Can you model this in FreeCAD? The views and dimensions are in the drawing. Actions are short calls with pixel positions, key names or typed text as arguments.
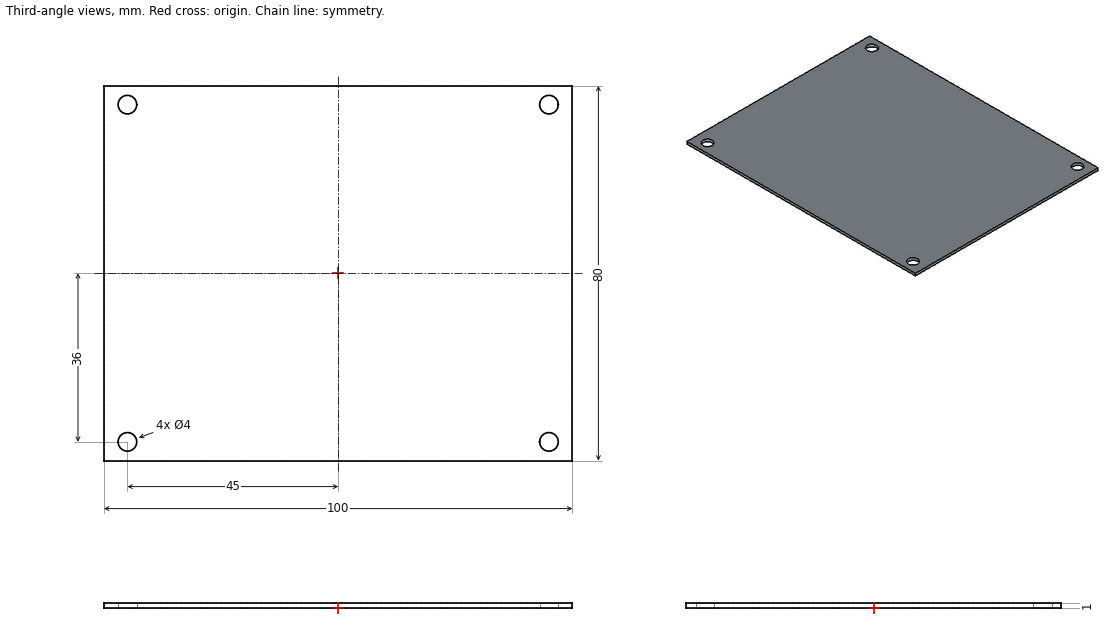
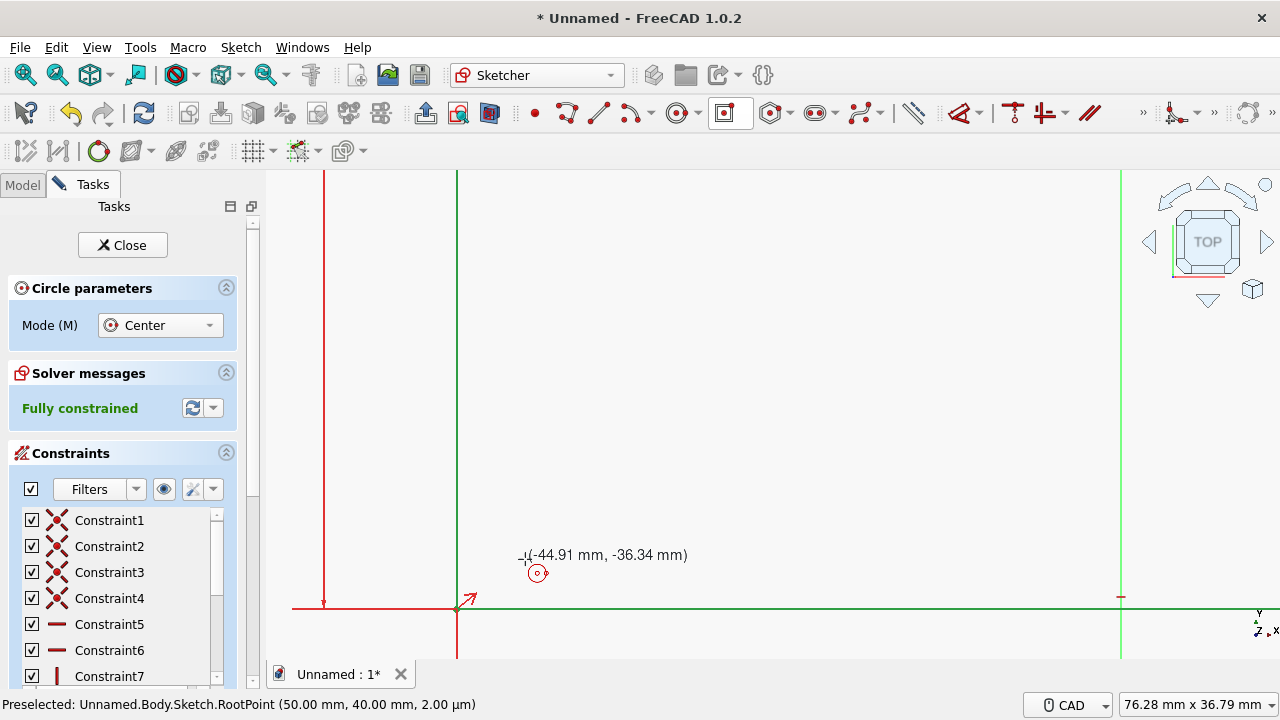
click(523, 556)
move(542, 537)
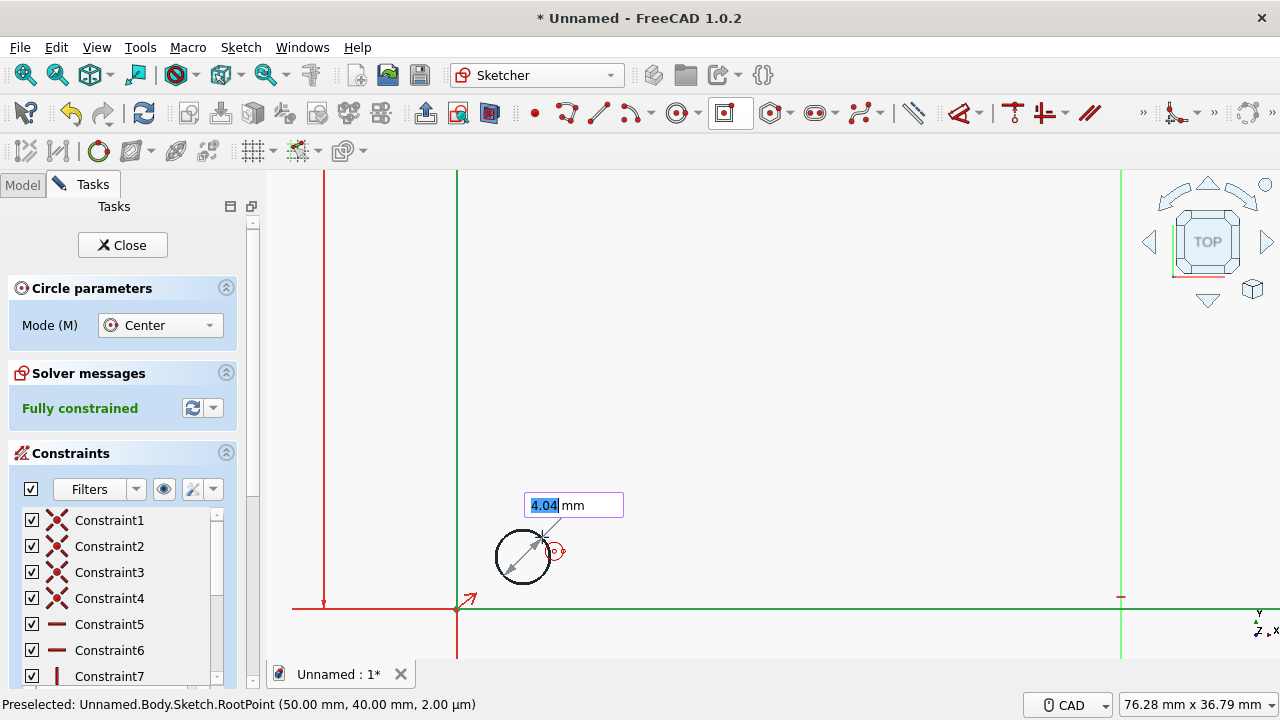
text(4)
key(Return)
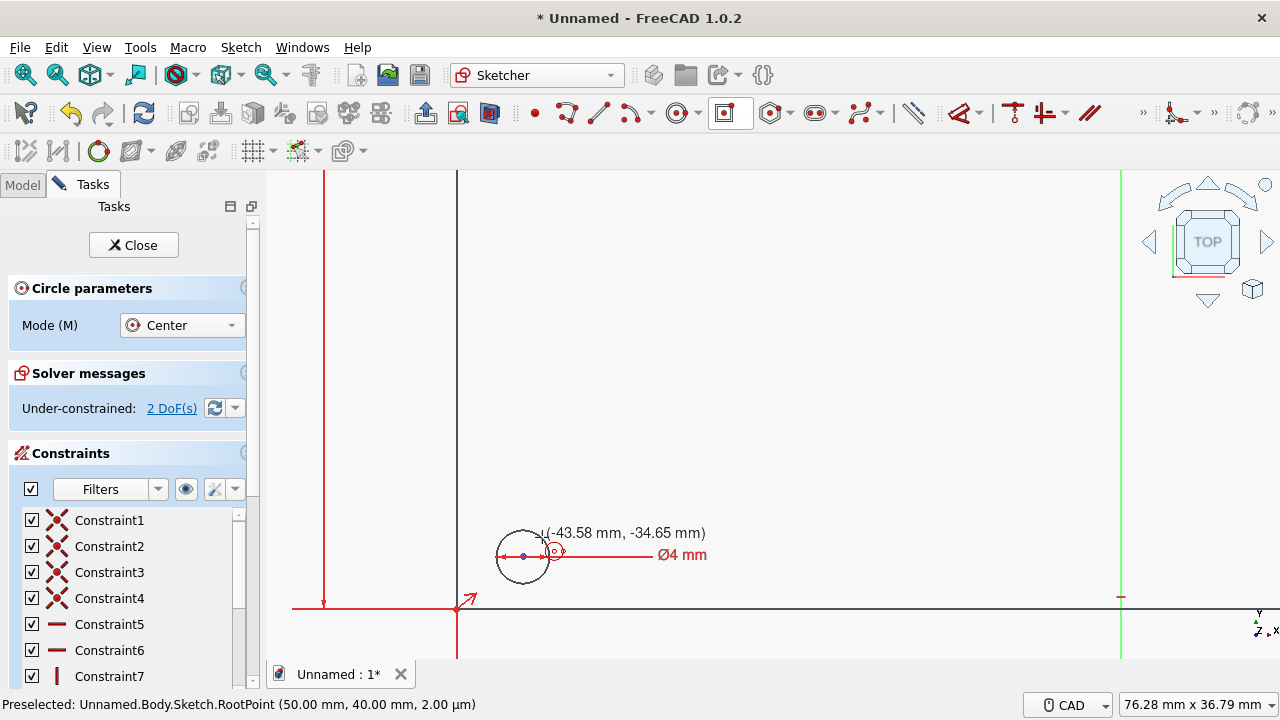
scroll(525, 560, down, 6)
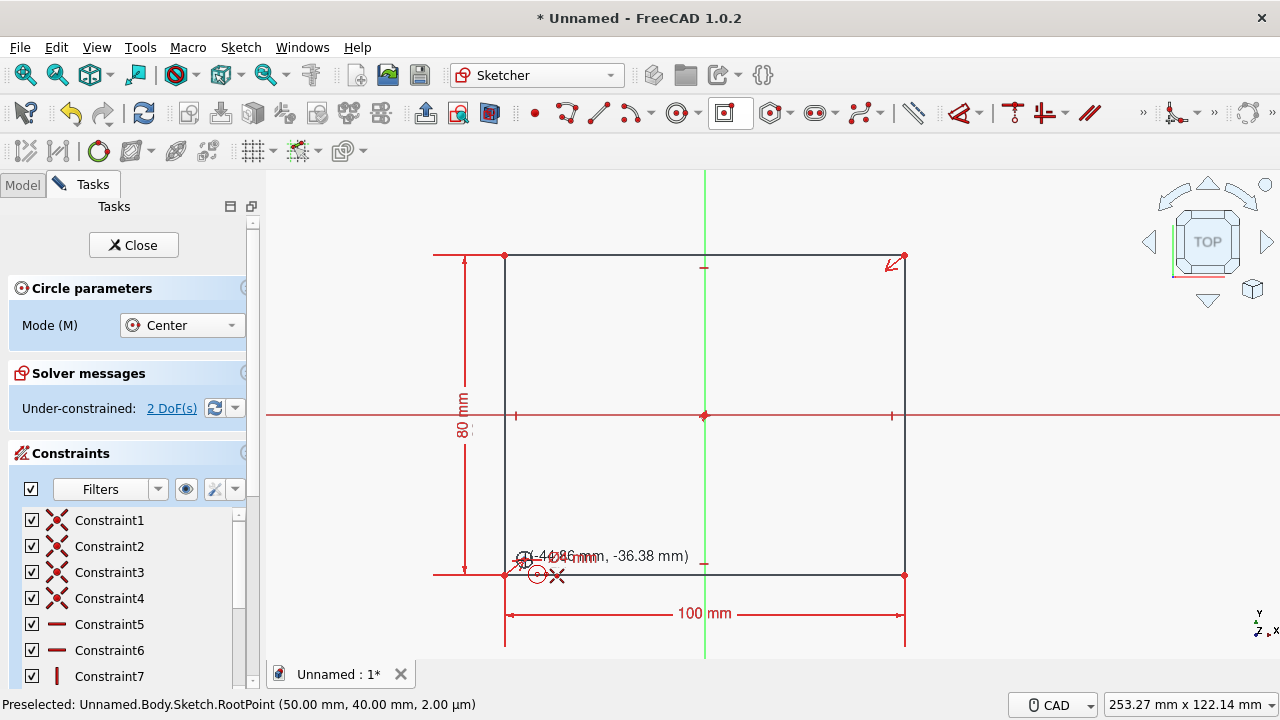
scroll(885, 559, up, 6)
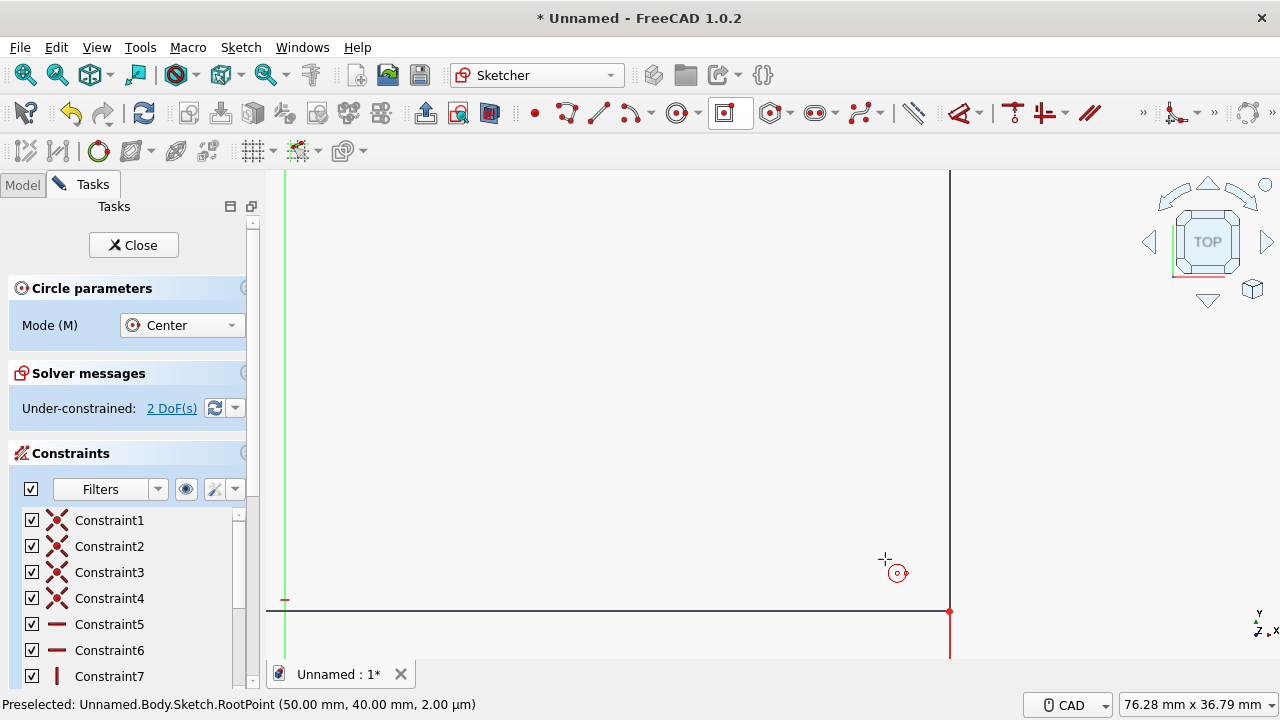
click(883, 558)
move(902, 539)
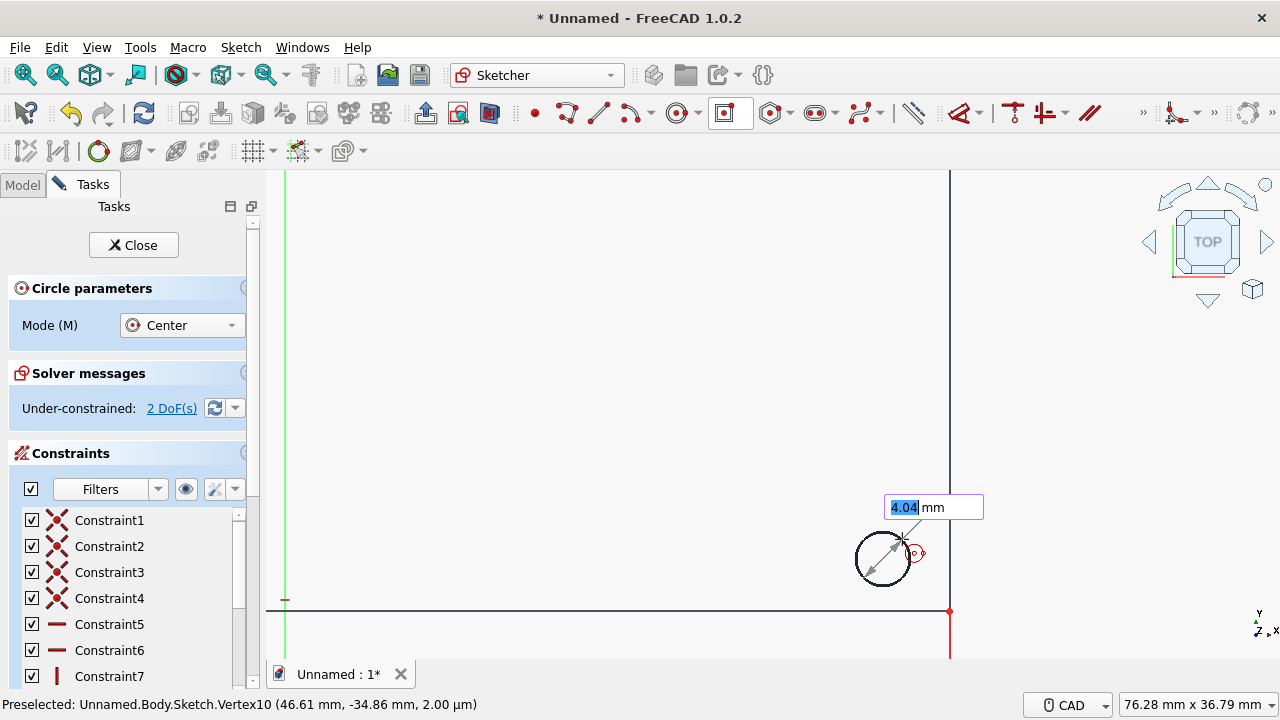
text(4)
key(Return)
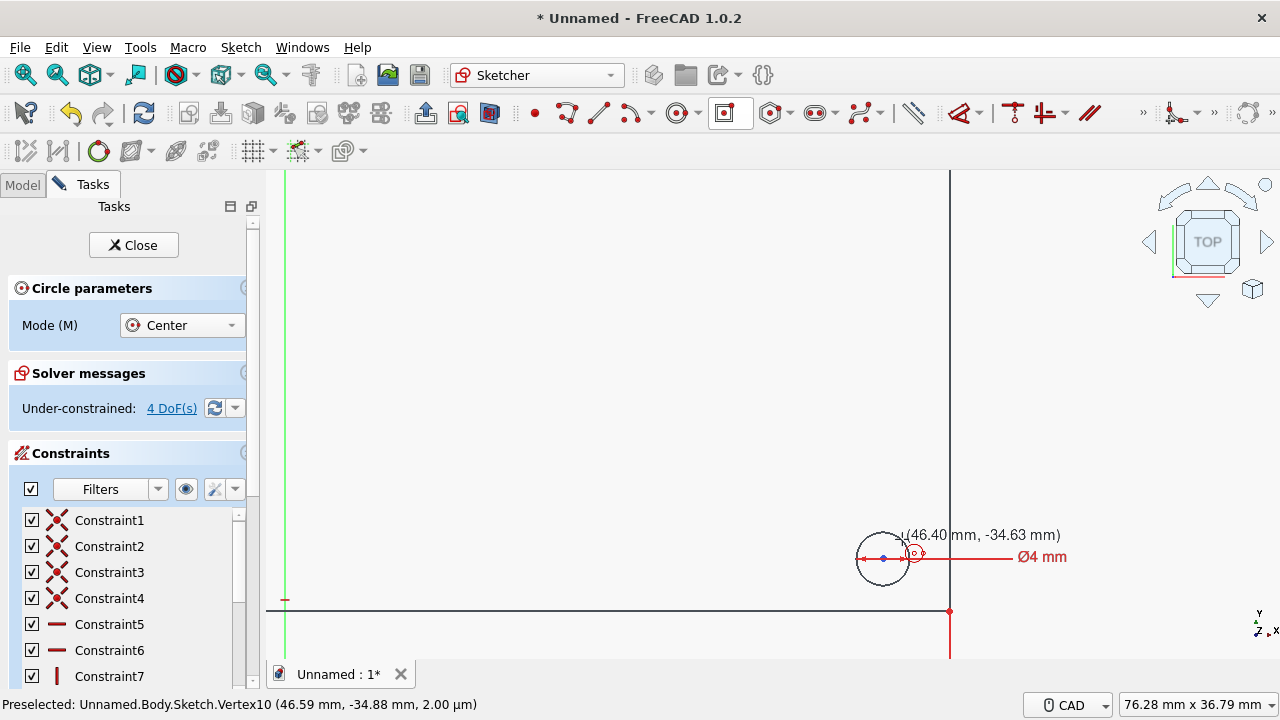
scroll(885, 559, down, 6)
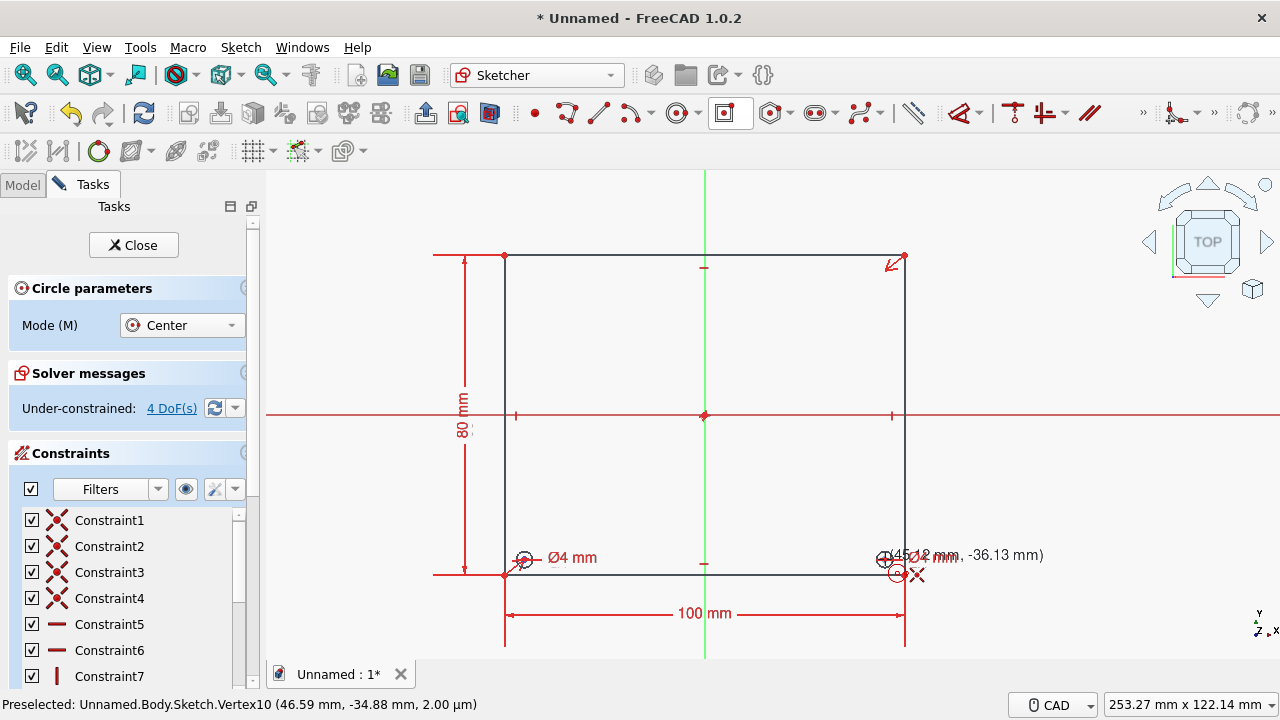
scroll(525, 271, up, 6)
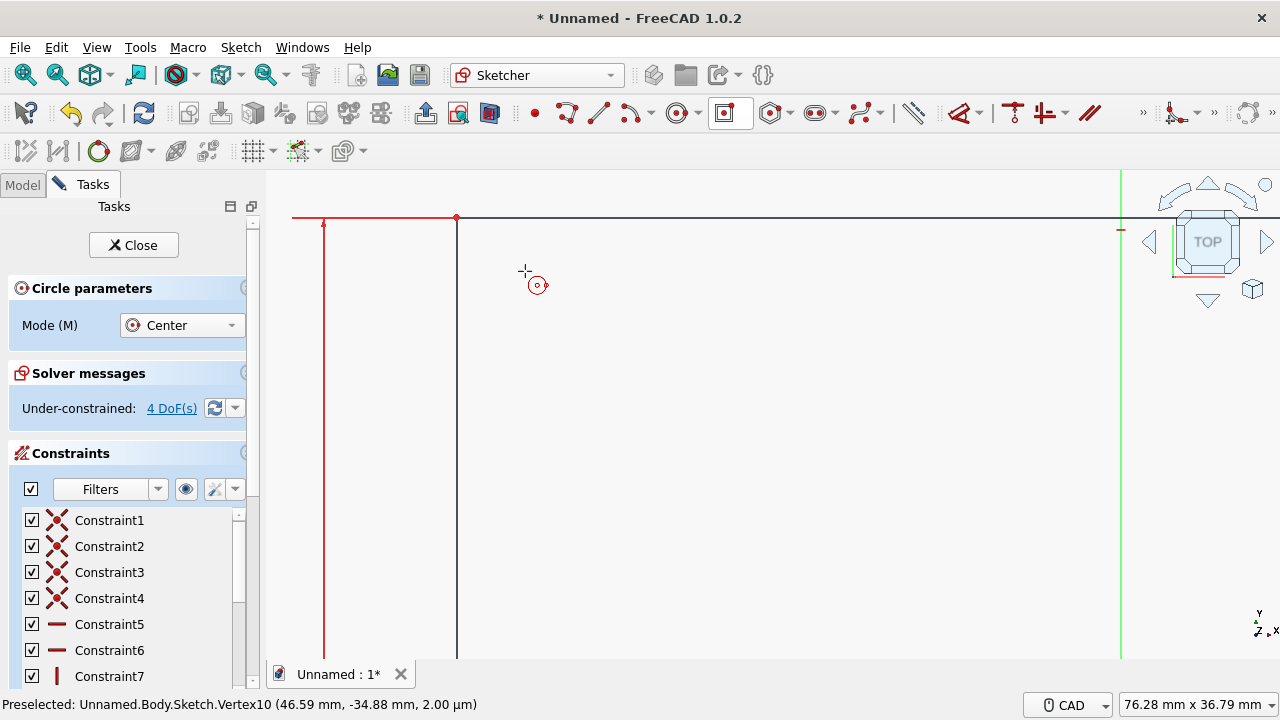
click(523, 271)
move(542, 252)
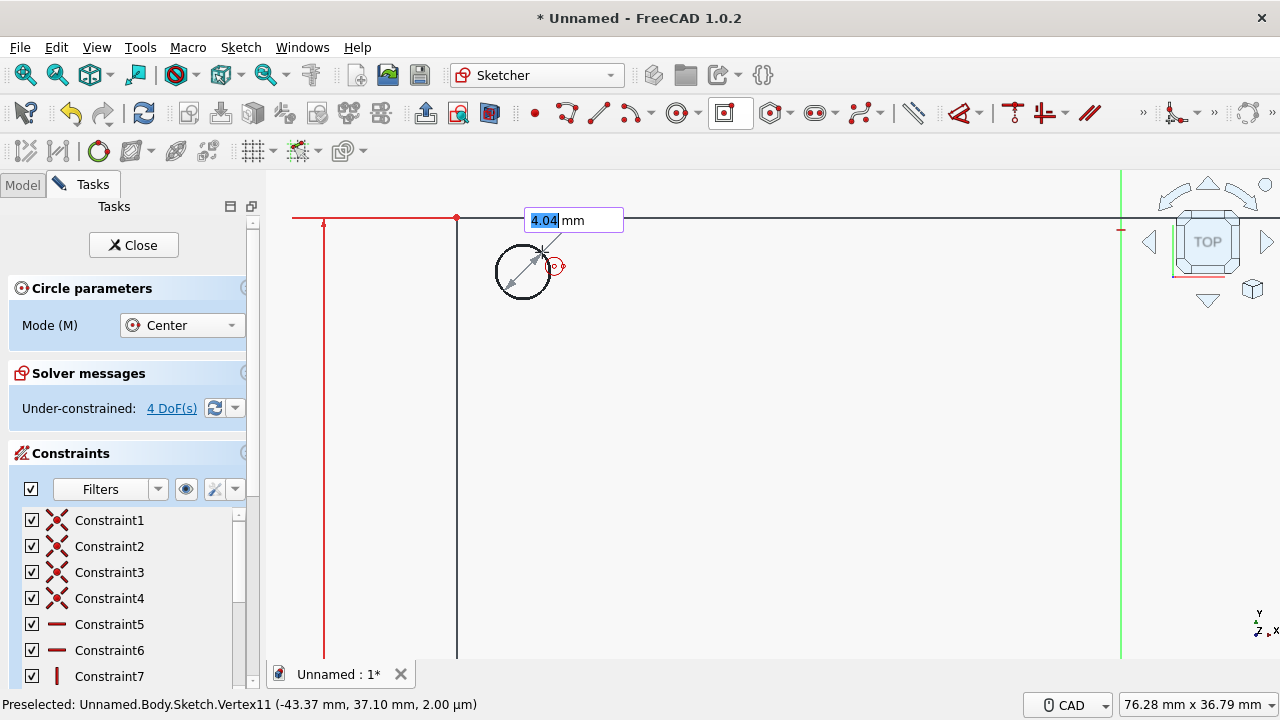
text(4)
key(Return)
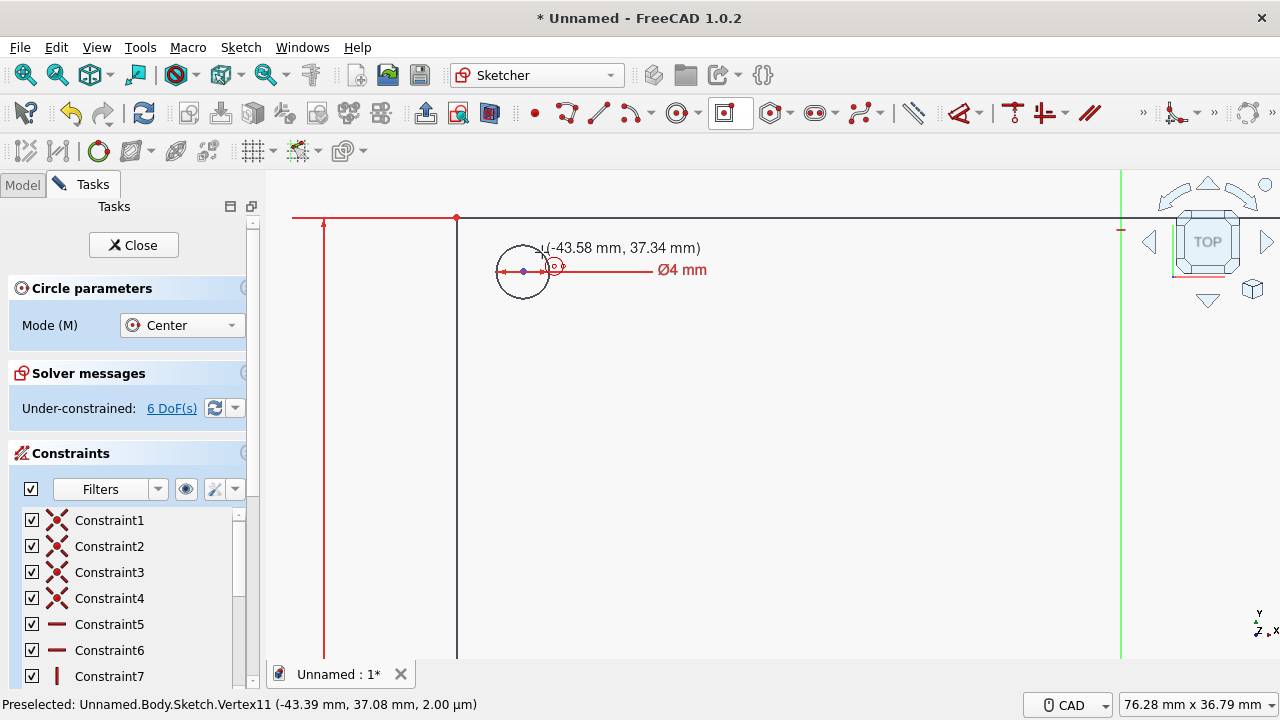
scroll(525, 270, down, 6)